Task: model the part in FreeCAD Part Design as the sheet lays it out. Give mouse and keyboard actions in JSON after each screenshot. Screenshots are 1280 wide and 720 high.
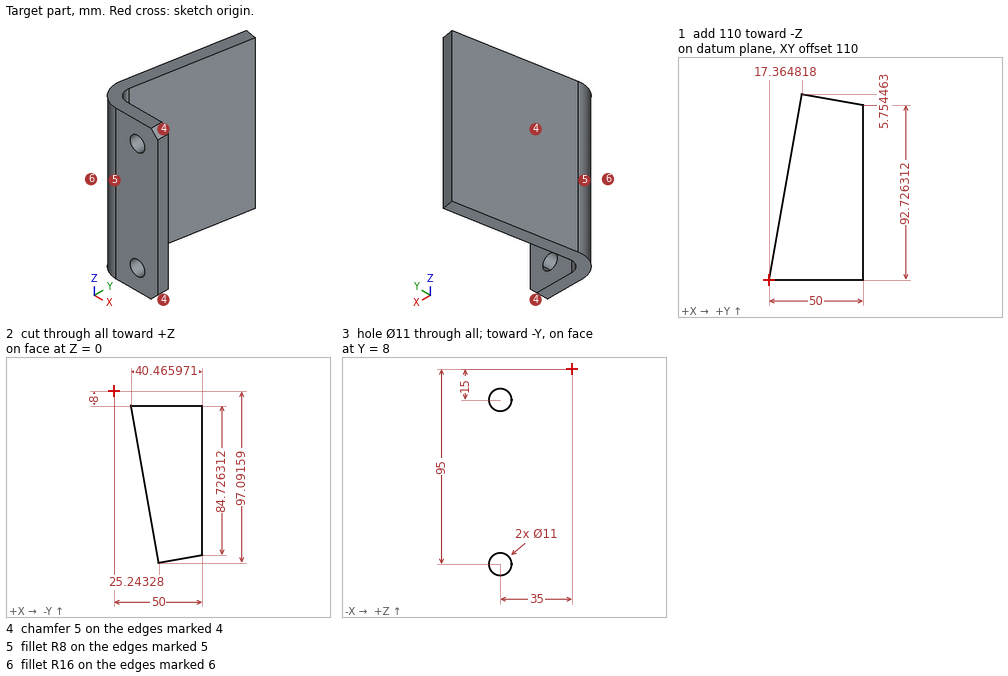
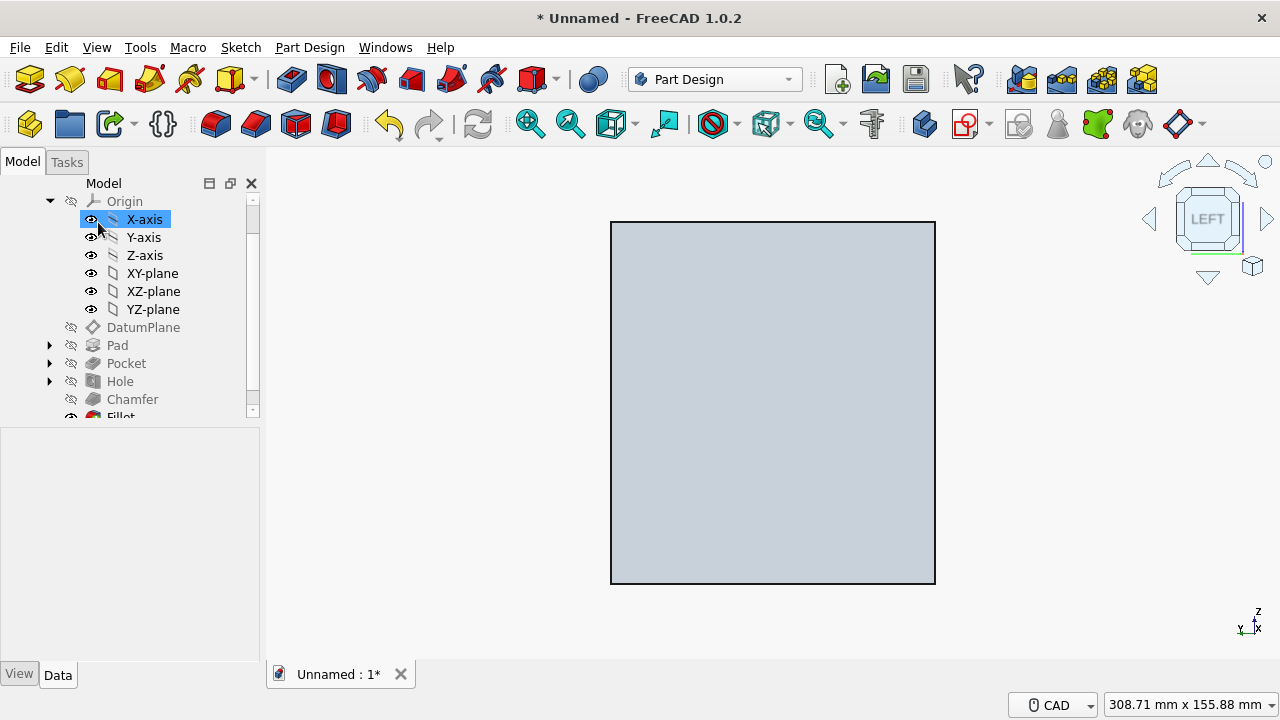
{"action": "left_click", "coordinate": [935, 402]}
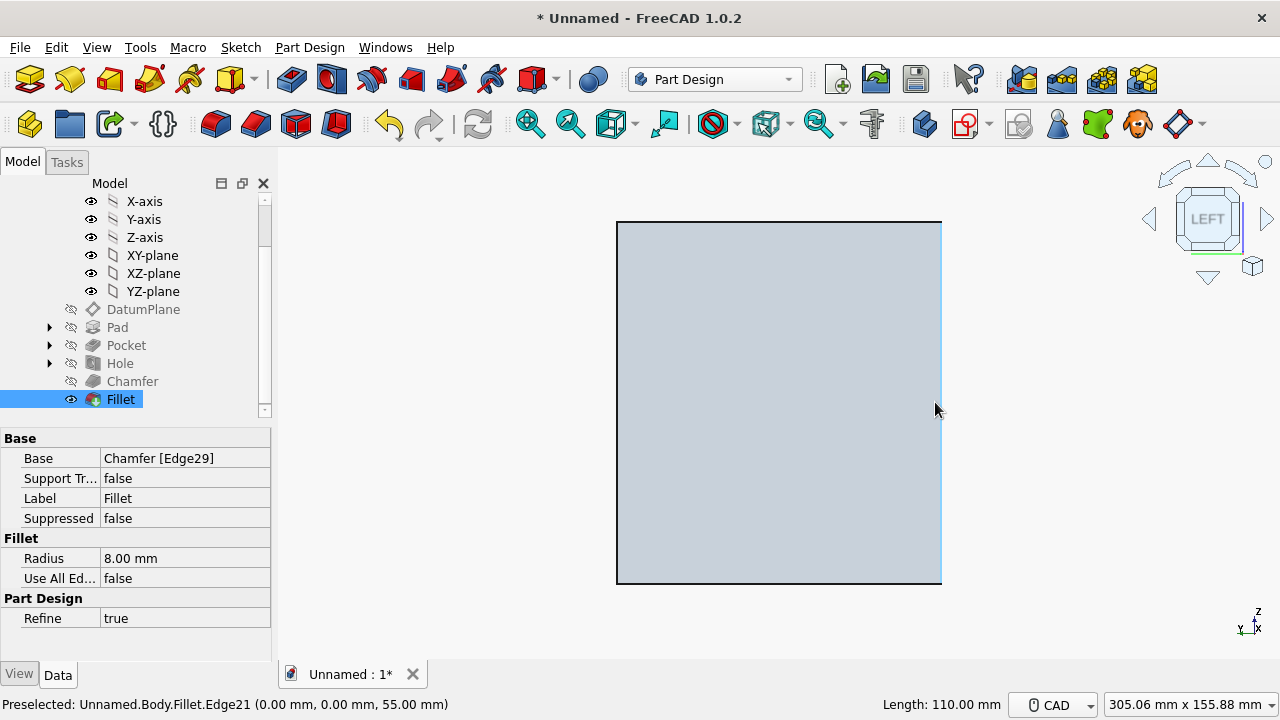
{"action": "left_click", "coordinate": [216, 124]}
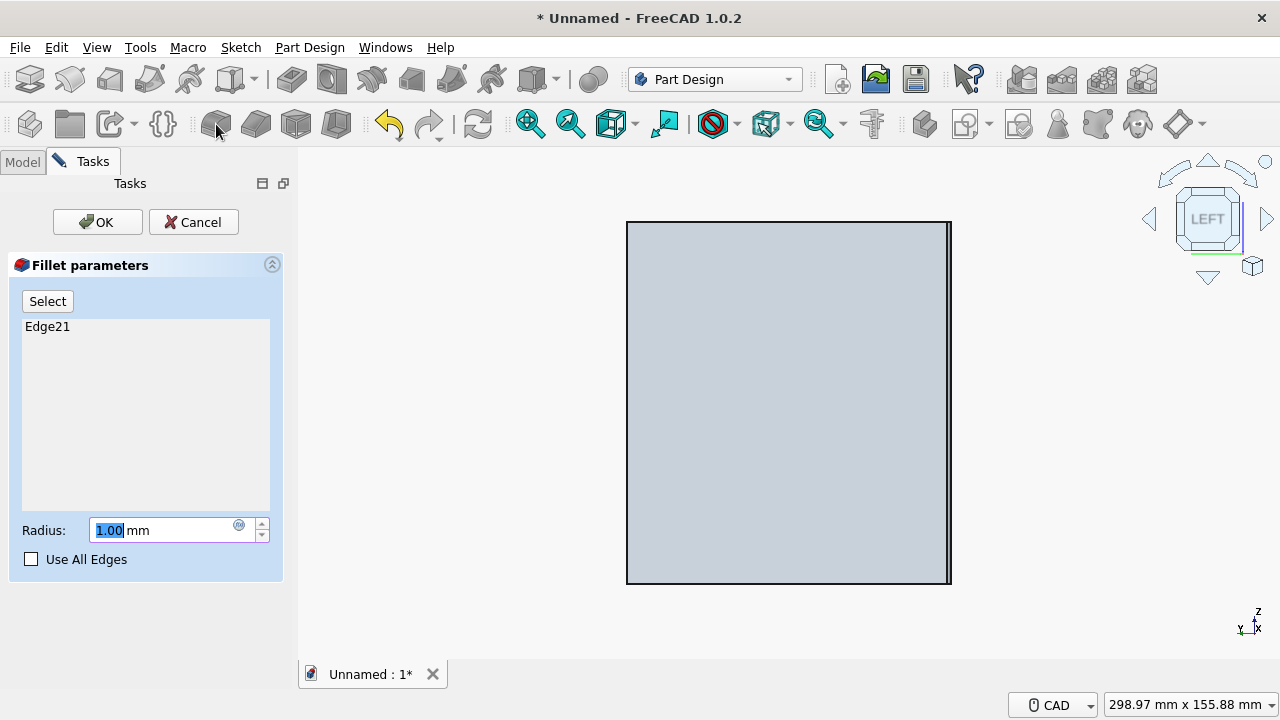
{"action": "type", "text": "16"}
{"action": "key", "text": "Tab"}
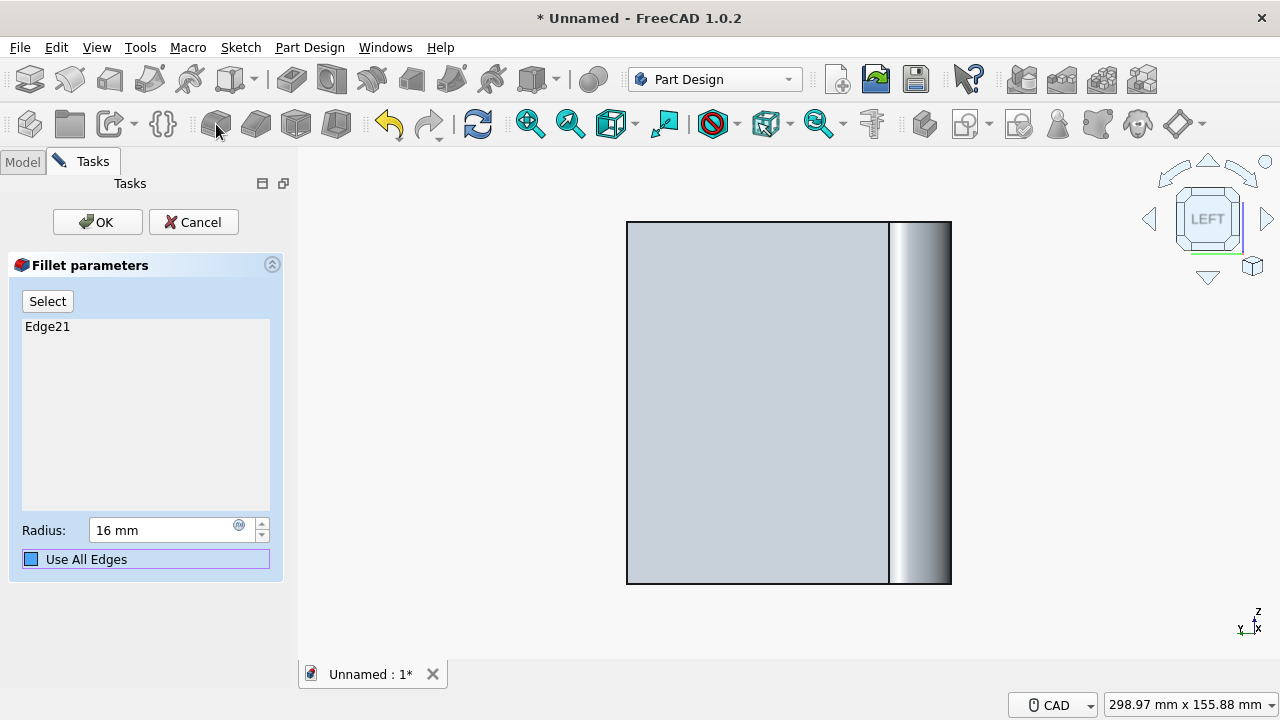
{"action": "left_click", "coordinate": [98, 222]}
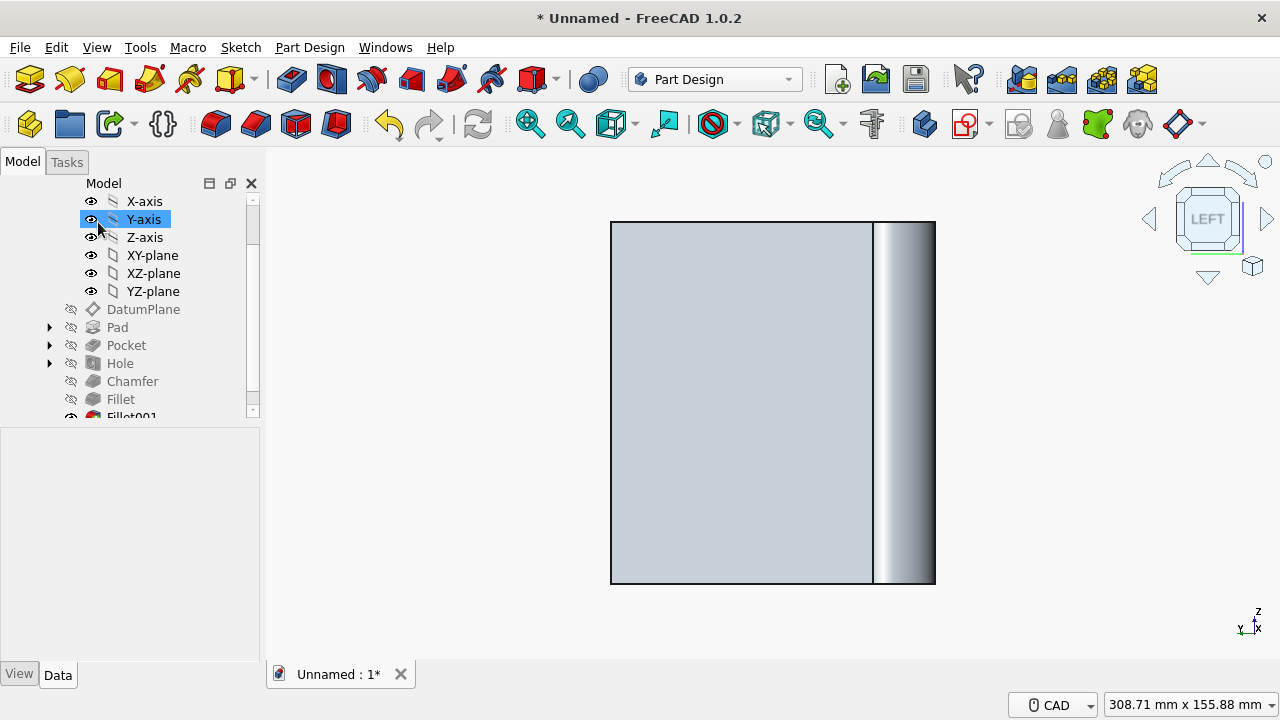
{"action": "key", "text": "0"}